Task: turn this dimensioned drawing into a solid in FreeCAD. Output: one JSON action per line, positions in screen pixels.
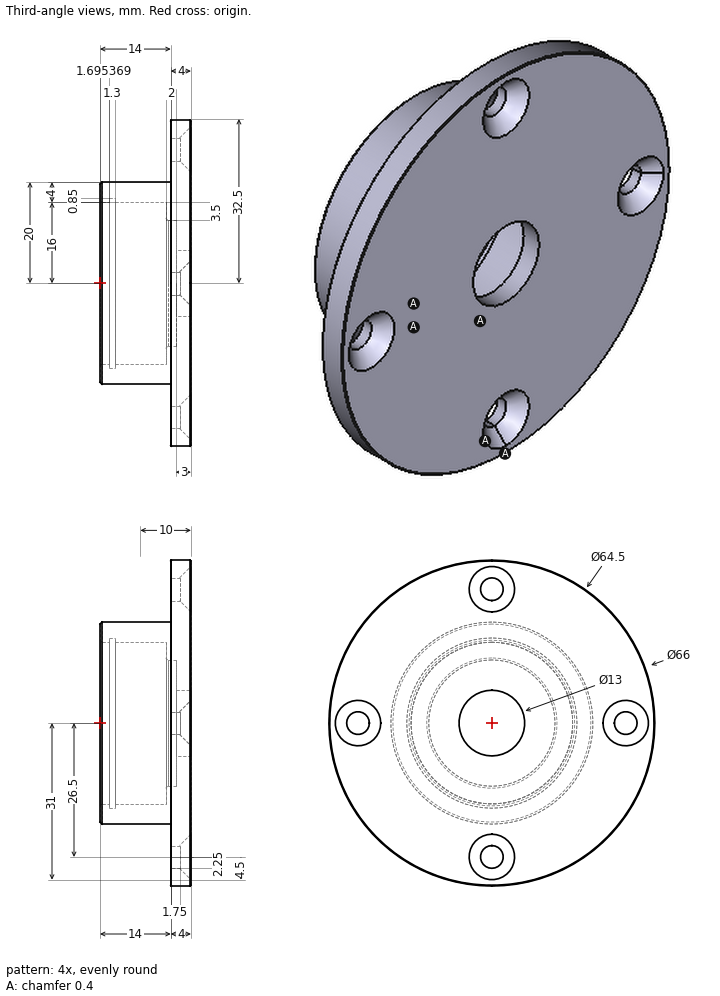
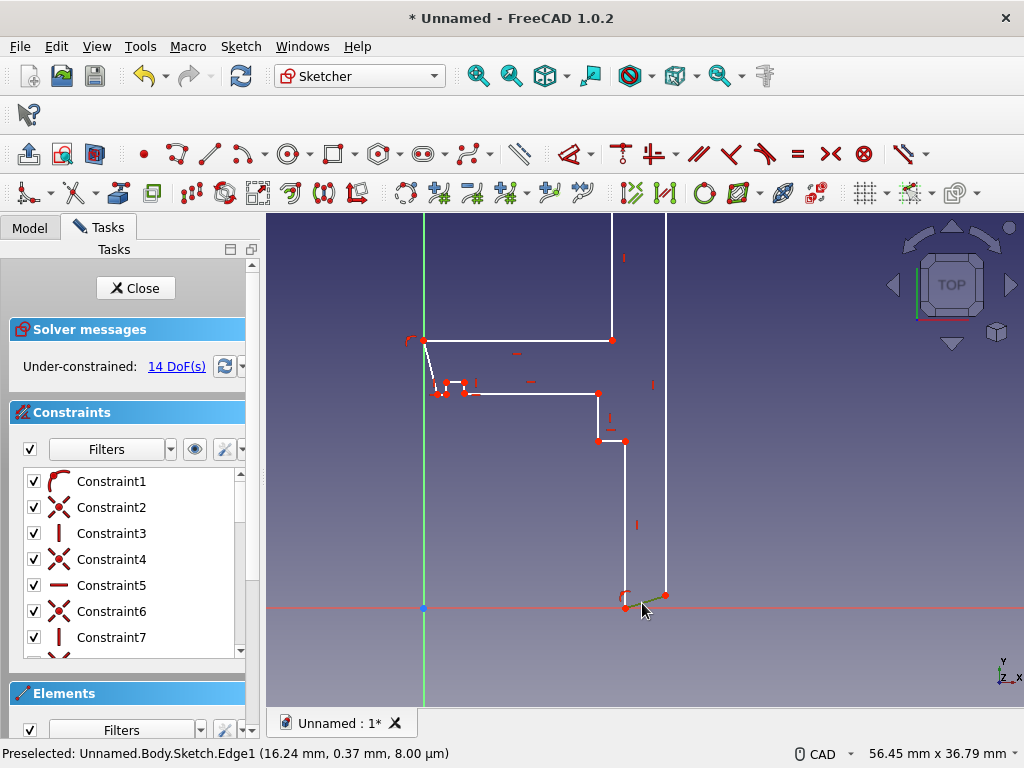
{"action": "left_click", "coordinate": [676, 154]}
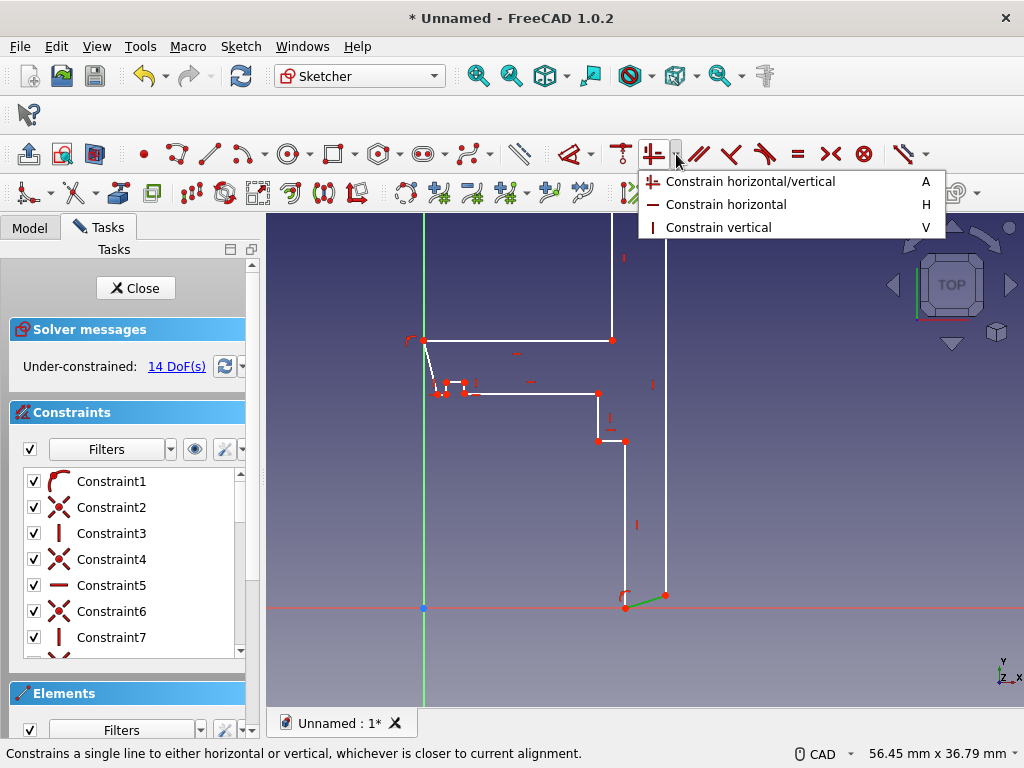
{"action": "left_click", "coordinate": [792, 204]}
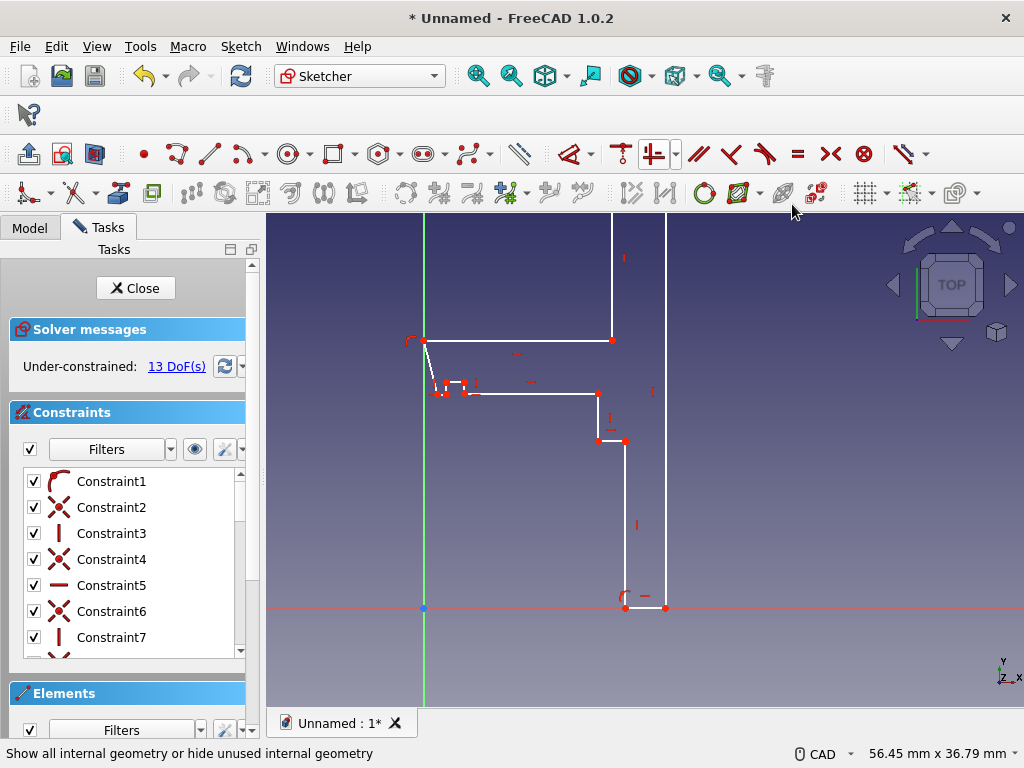
{"action": "scroll", "coordinate": [433, 378], "scroll_direction": "up", "scroll_amount": 2}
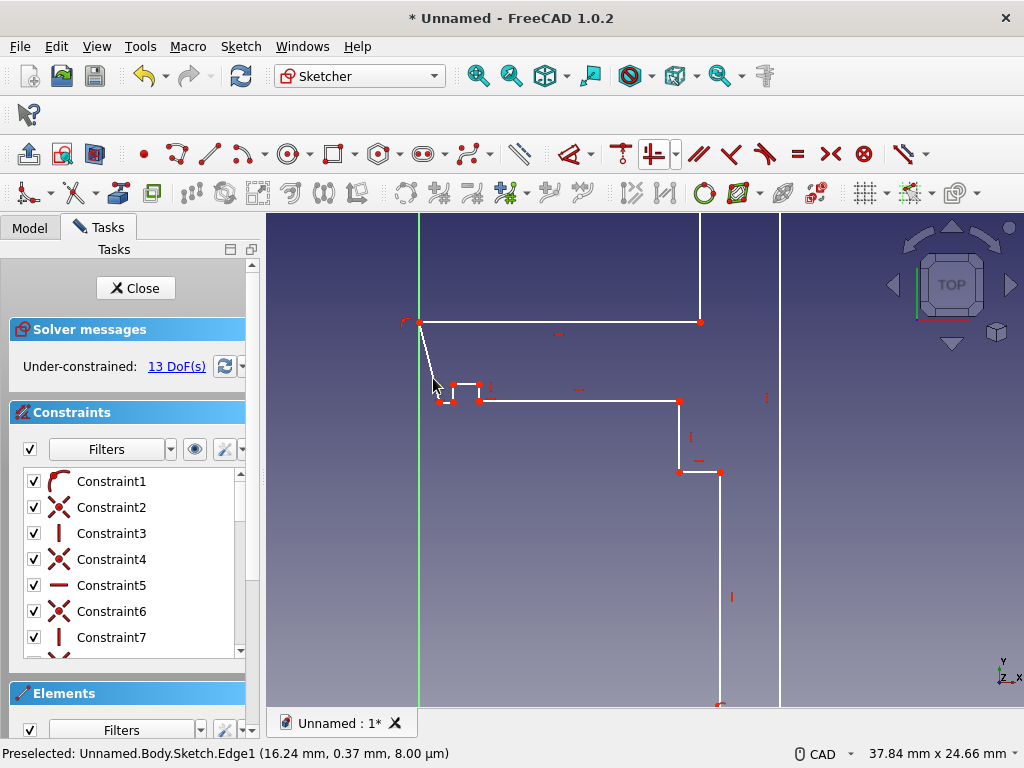
{"action": "left_click", "coordinate": [433, 379]}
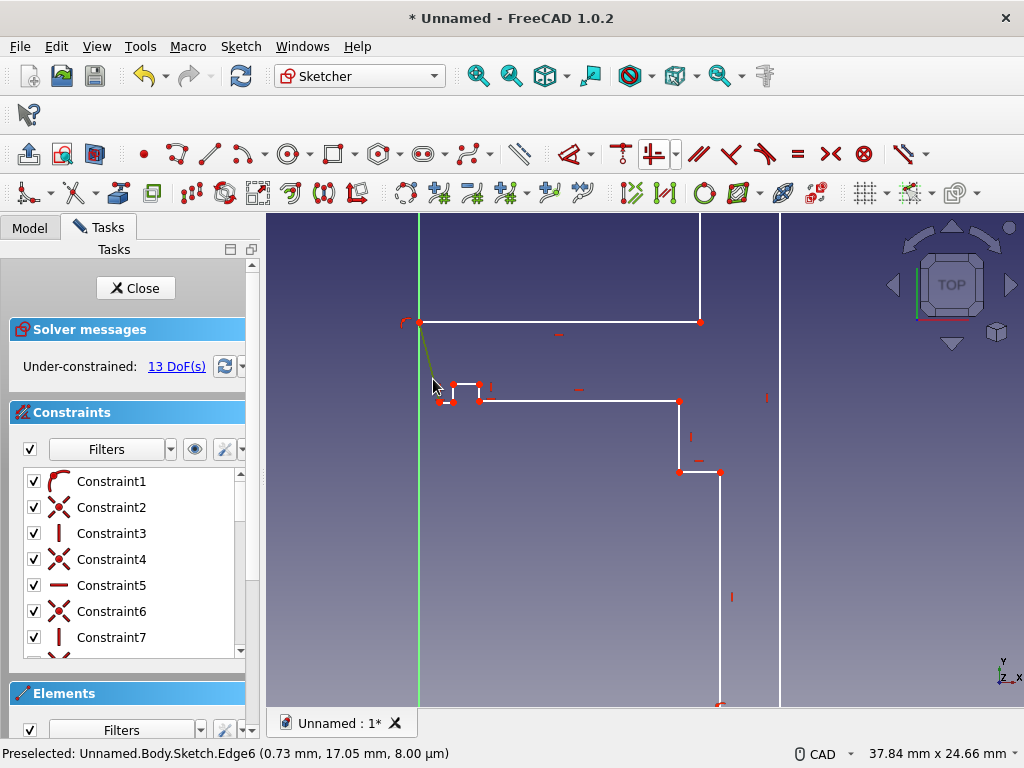
{"action": "key", "text": "v"}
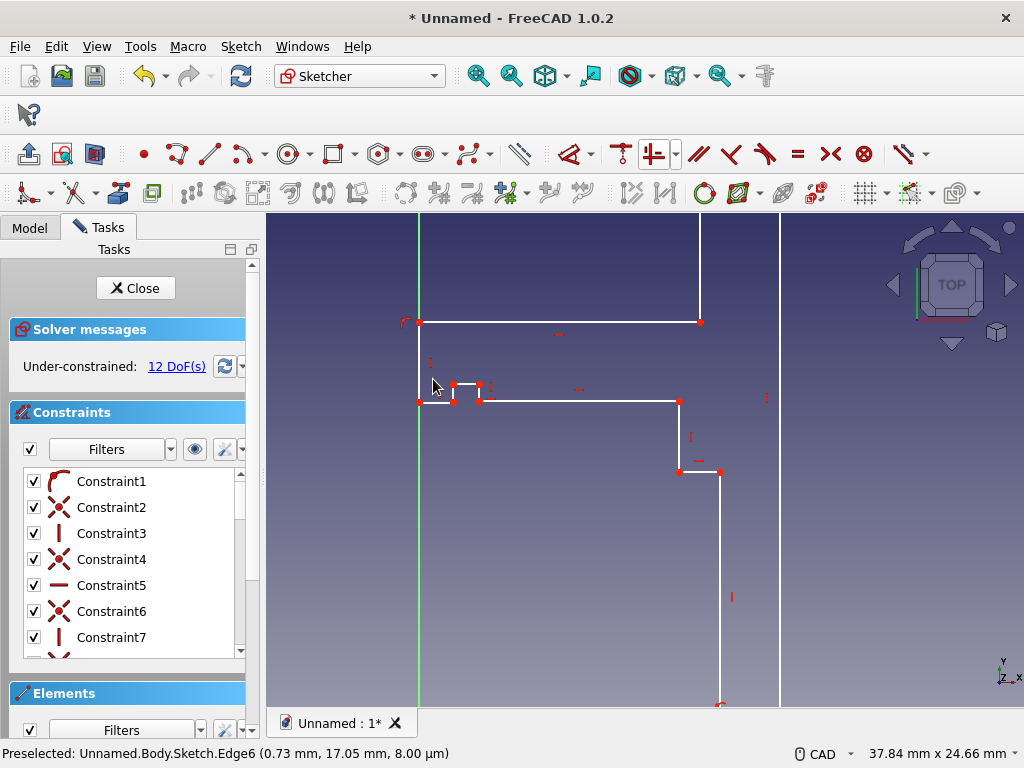
{"action": "scroll", "coordinate": [558, 512], "scroll_direction": "down", "scroll_amount": 4}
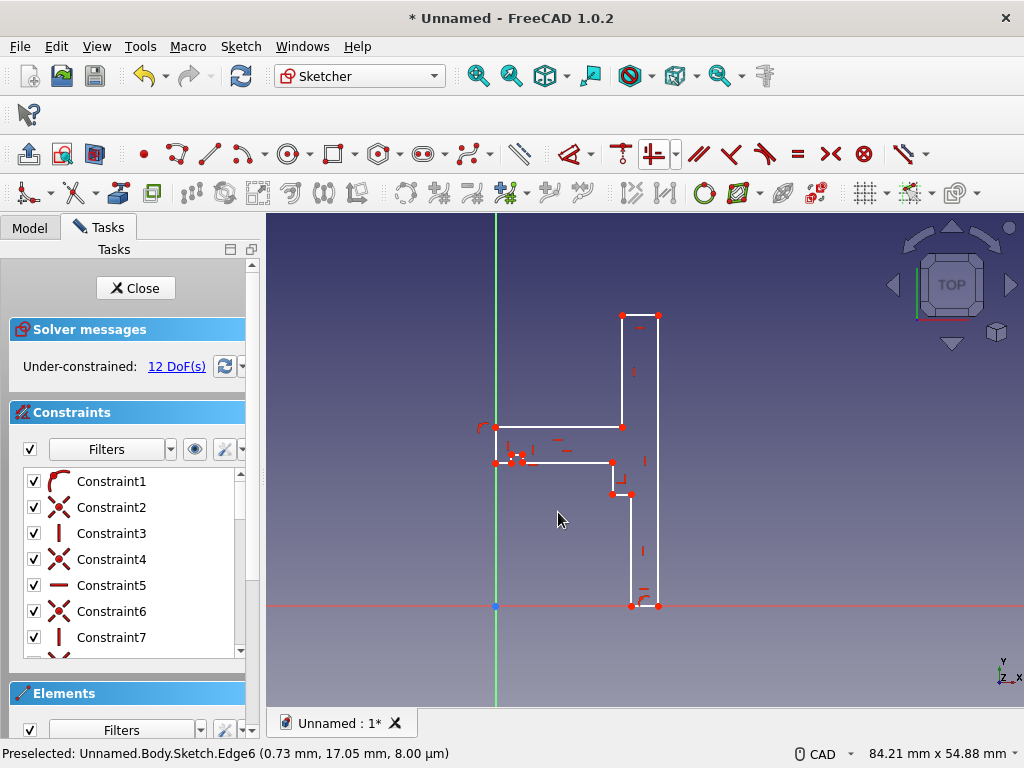
{"action": "scroll", "coordinate": [639, 606], "scroll_direction": "up", "scroll_amount": 3}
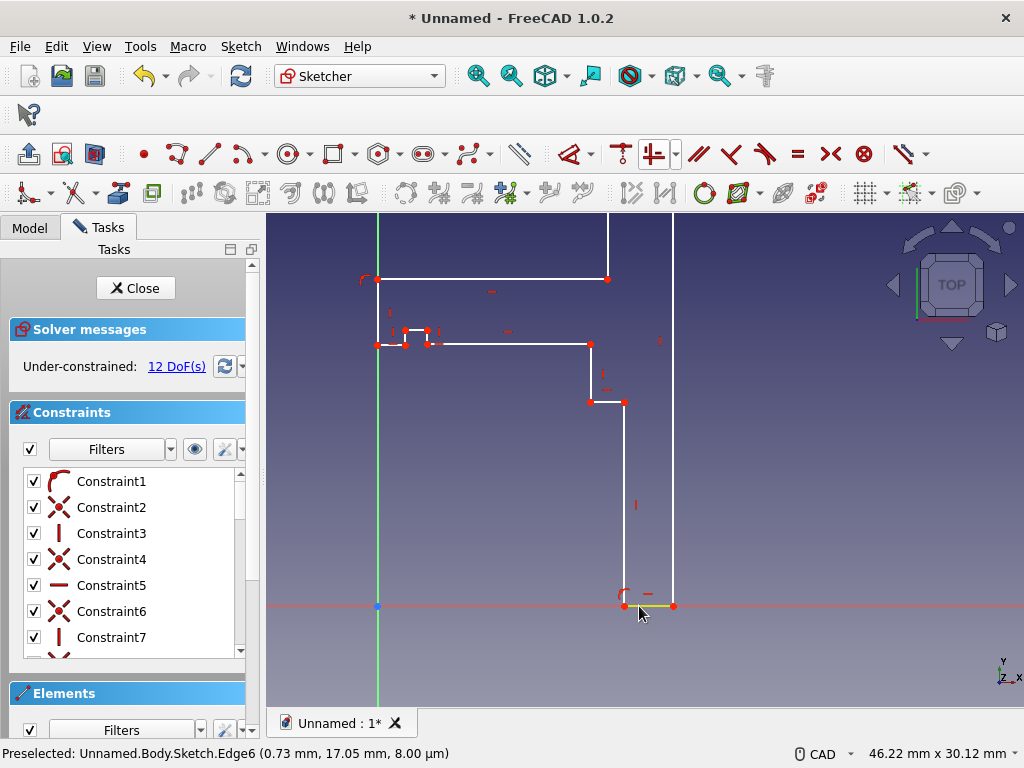
{"action": "left_click", "coordinate": [639, 606]}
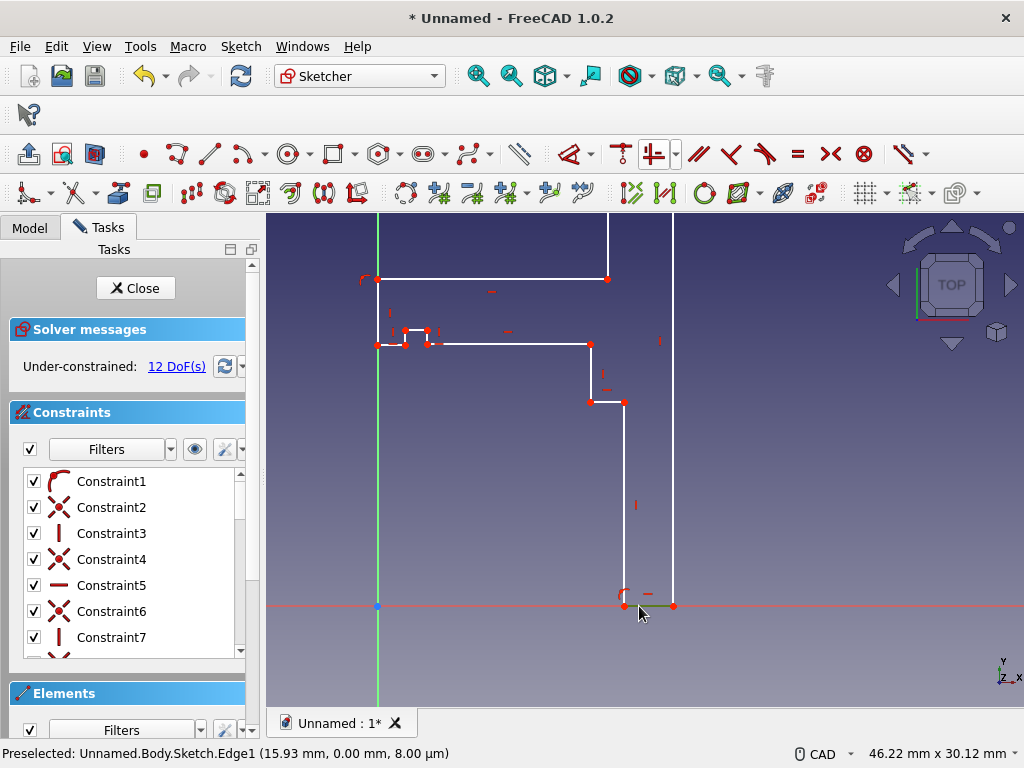
{"action": "left_click", "coordinate": [590, 154]}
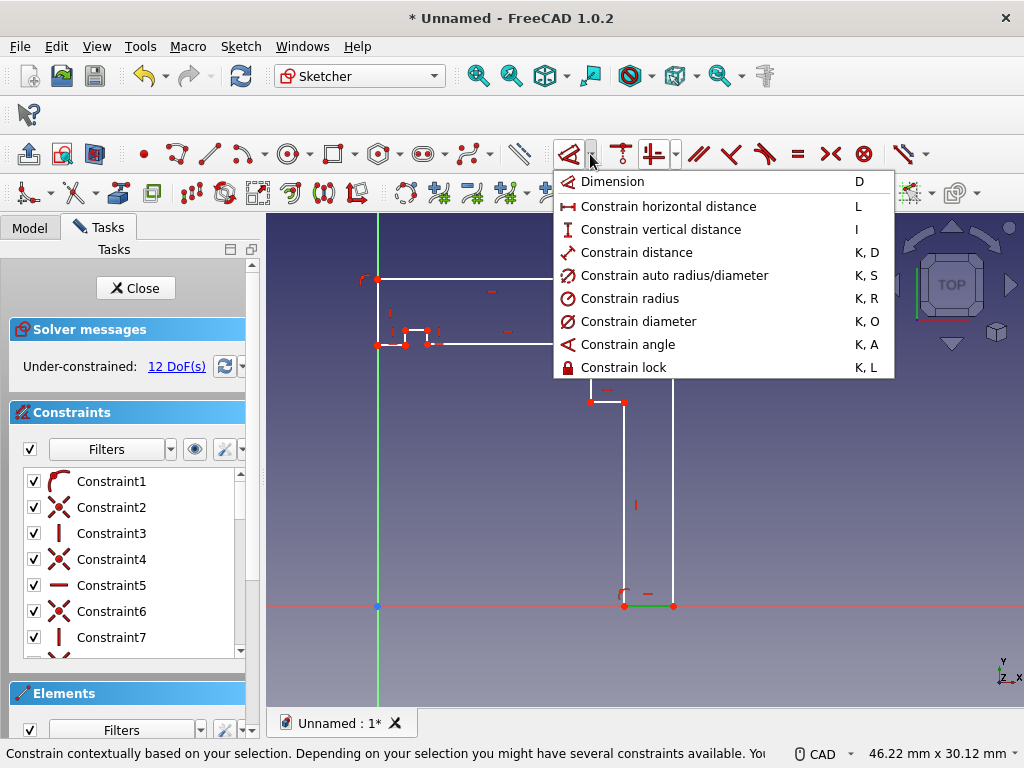
{"action": "left_click", "coordinate": [724, 206]}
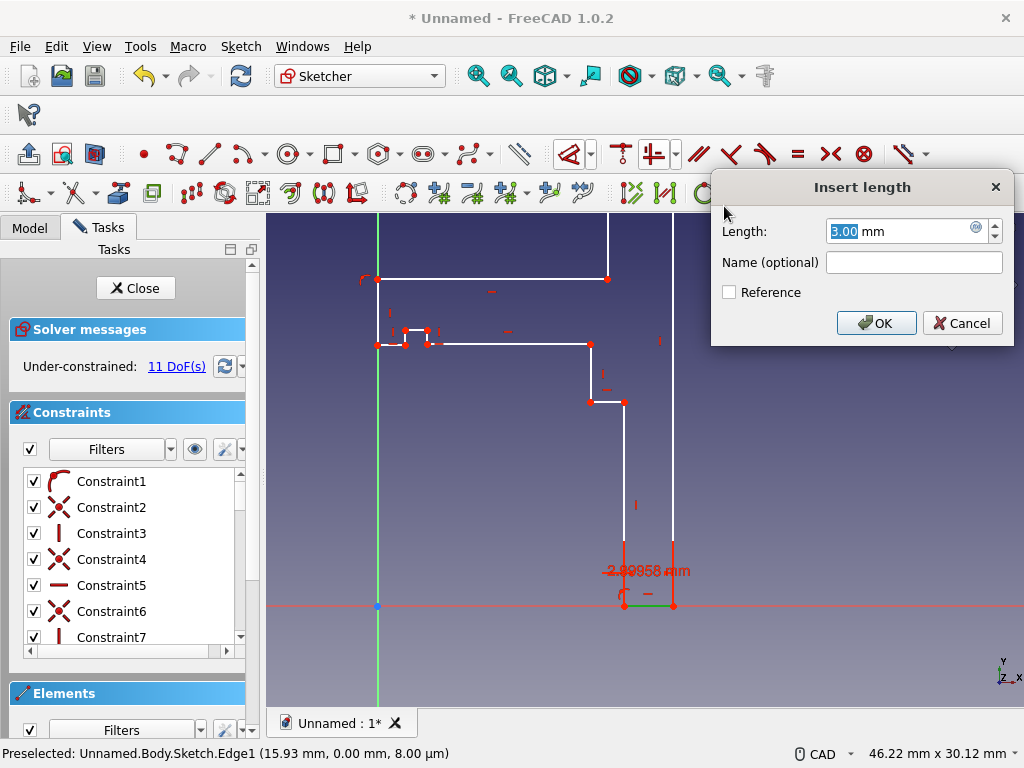
{"action": "type", "text": "3"}
{"action": "key", "text": "Return"}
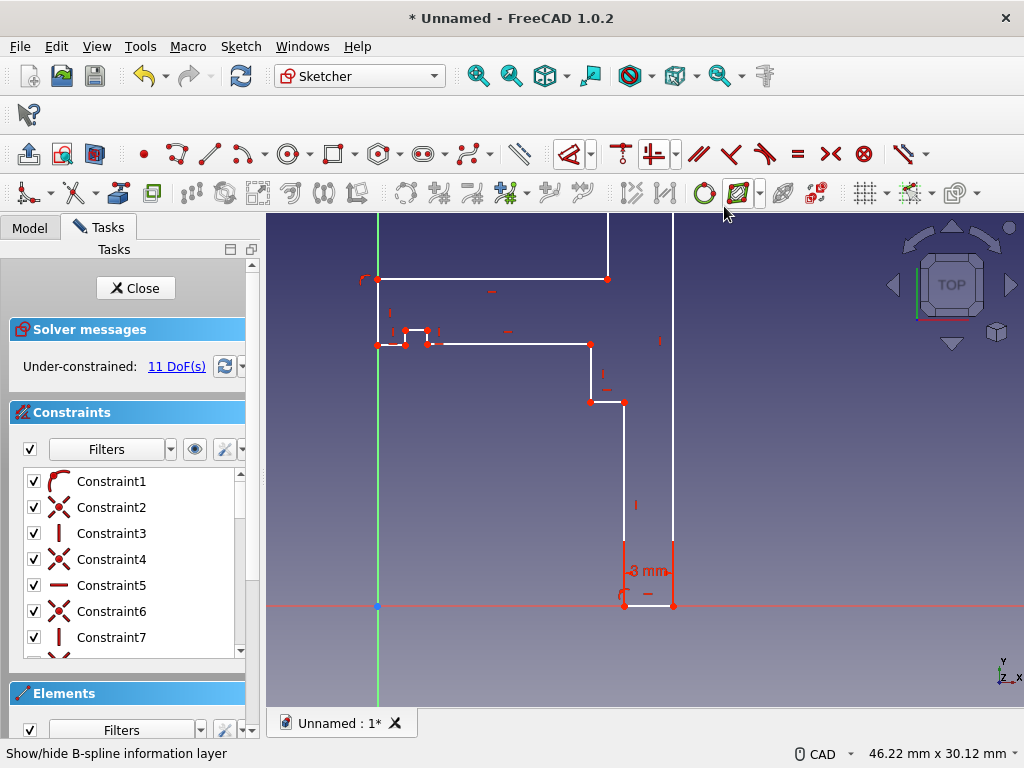
{"action": "scroll", "coordinate": [639, 607], "scroll_direction": "down", "scroll_amount": 3}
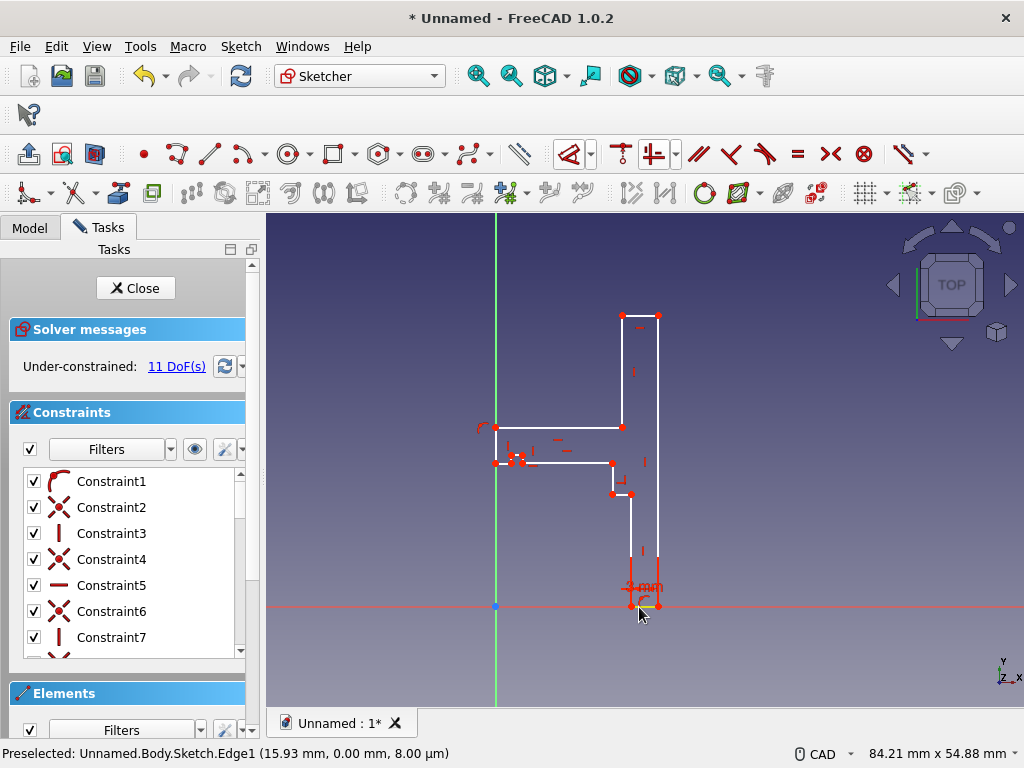
{"action": "scroll", "coordinate": [647, 316], "scroll_direction": "up", "scroll_amount": 2}